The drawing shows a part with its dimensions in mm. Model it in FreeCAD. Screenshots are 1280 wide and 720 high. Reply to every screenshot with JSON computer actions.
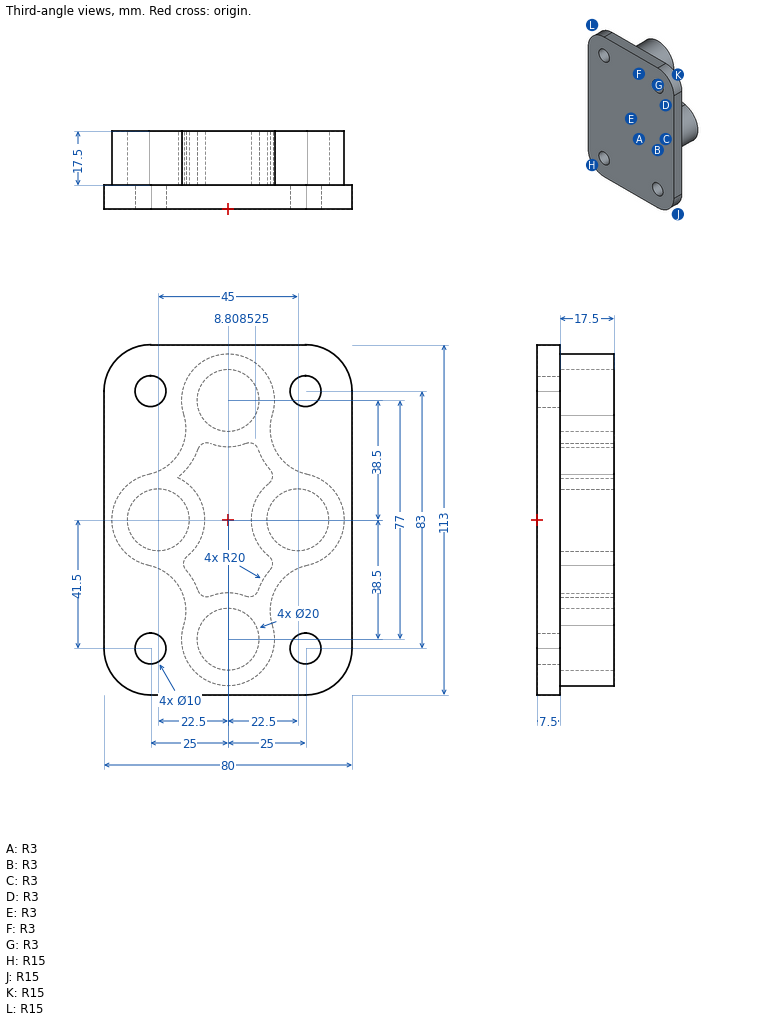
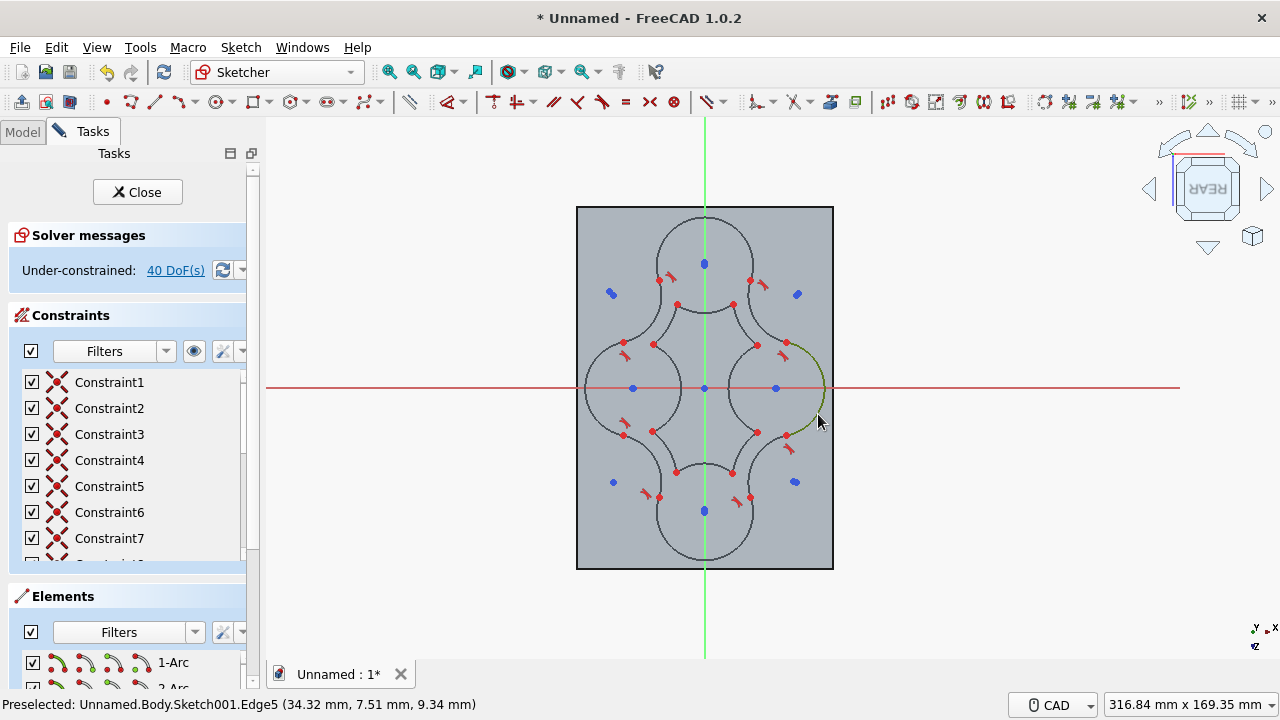
{"action": "left_click", "coordinate": [734, 368]}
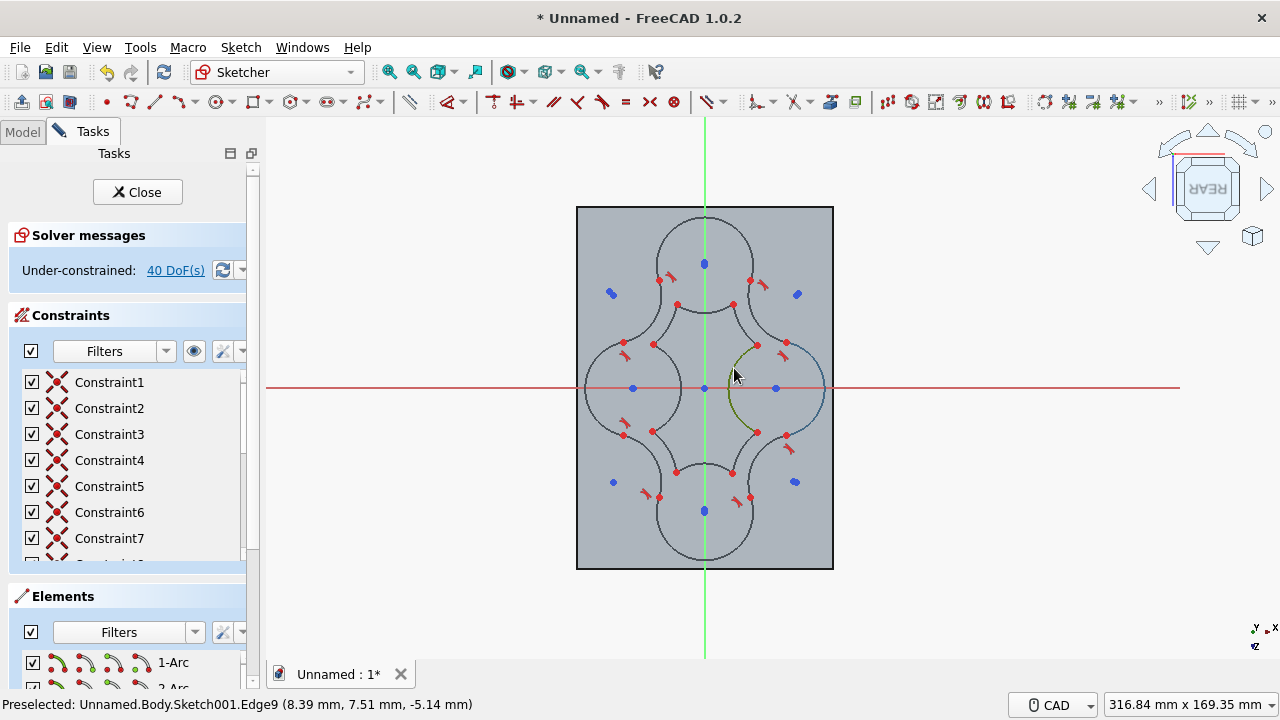
{"action": "key", "text": "c"}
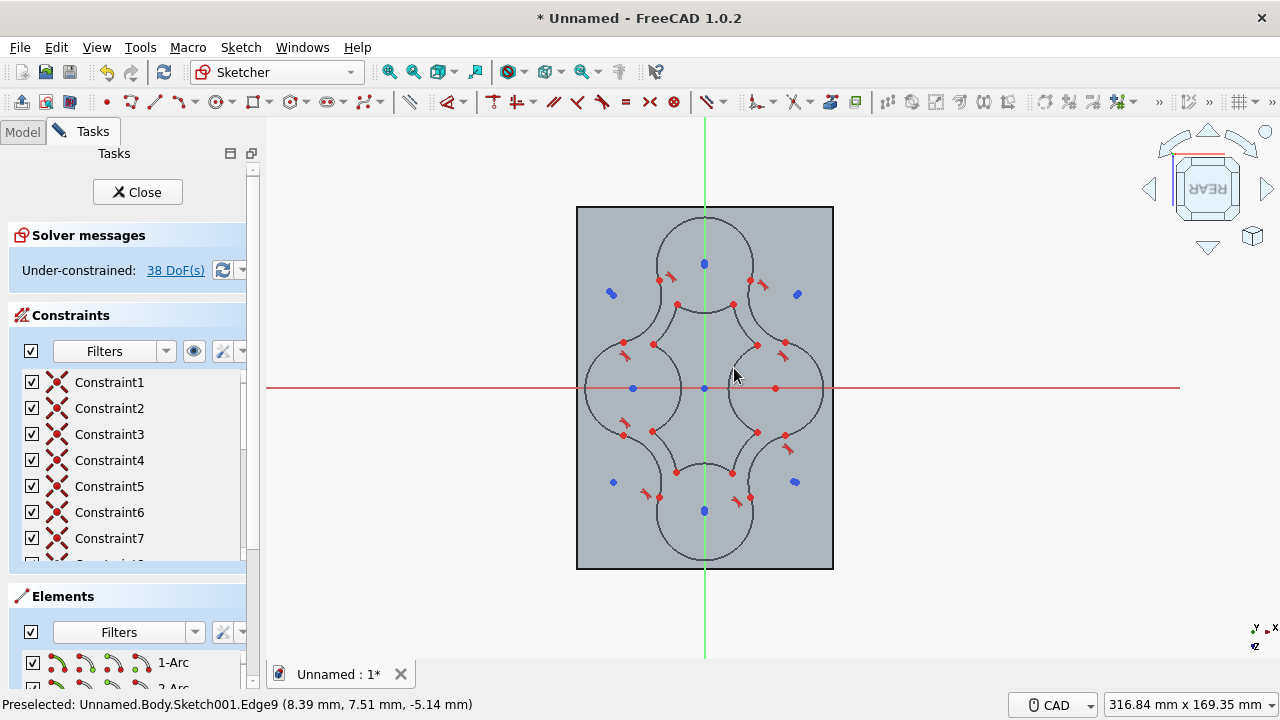
{"action": "left_click", "coordinate": [765, 446]}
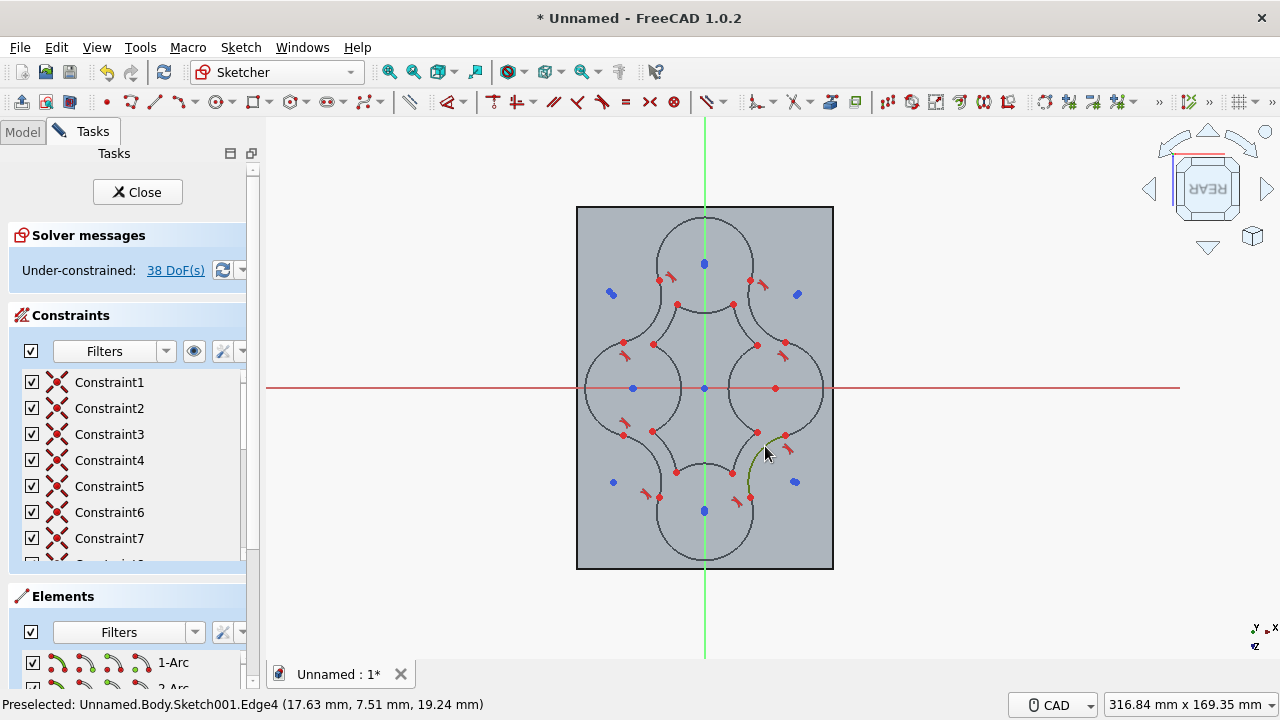
{"action": "left_click", "coordinate": [747, 442]}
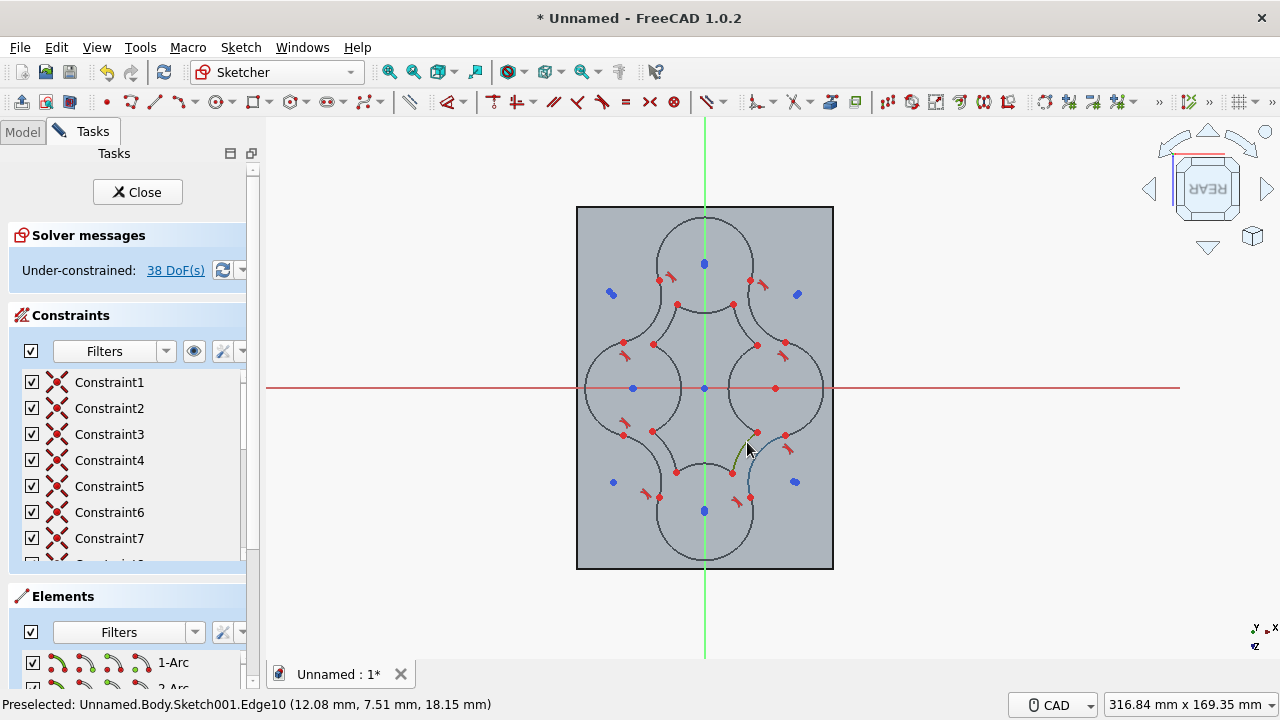
{"action": "key", "text": "c"}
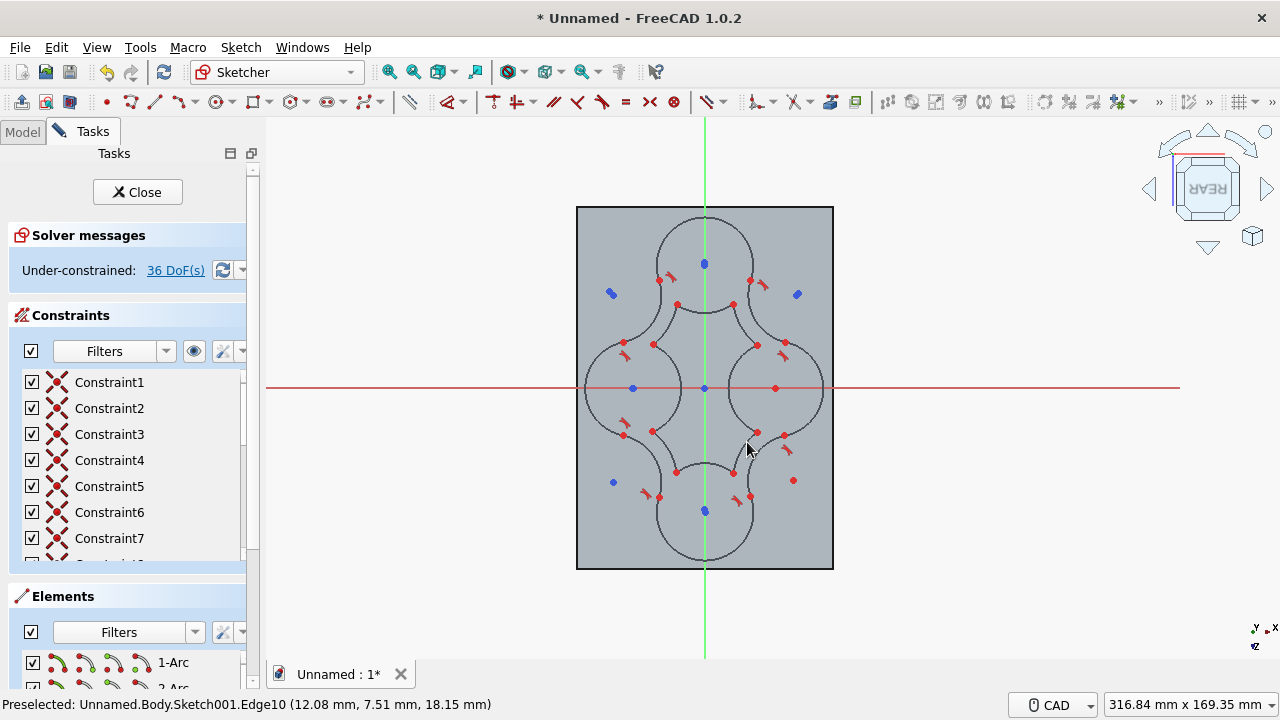
{"action": "left_click", "coordinate": [672, 548]}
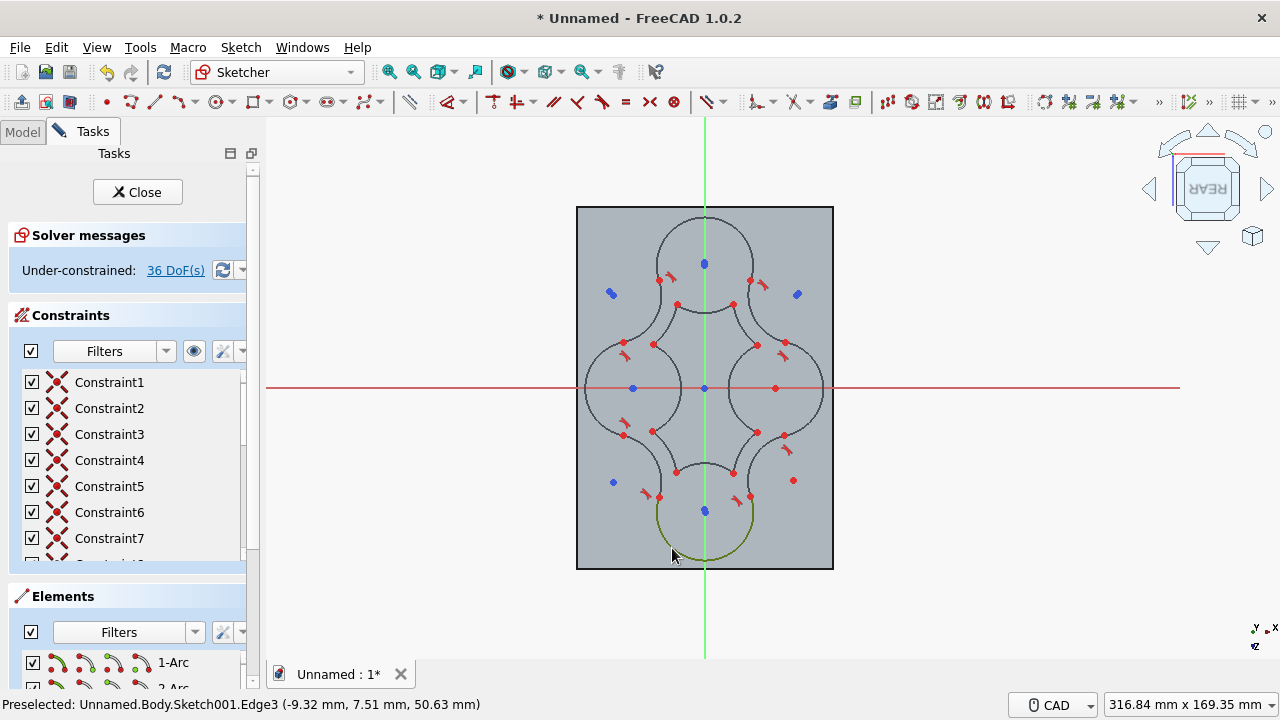
{"action": "left_click", "coordinate": [717, 465]}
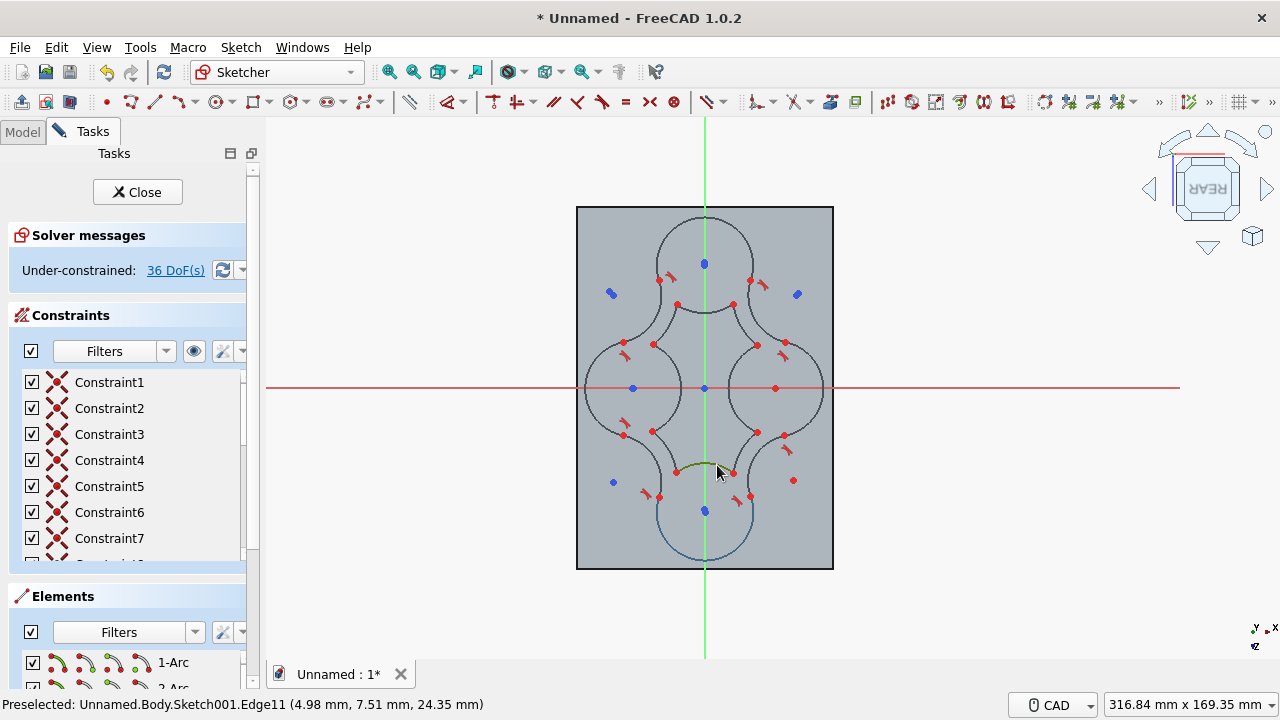
{"action": "key", "text": "c"}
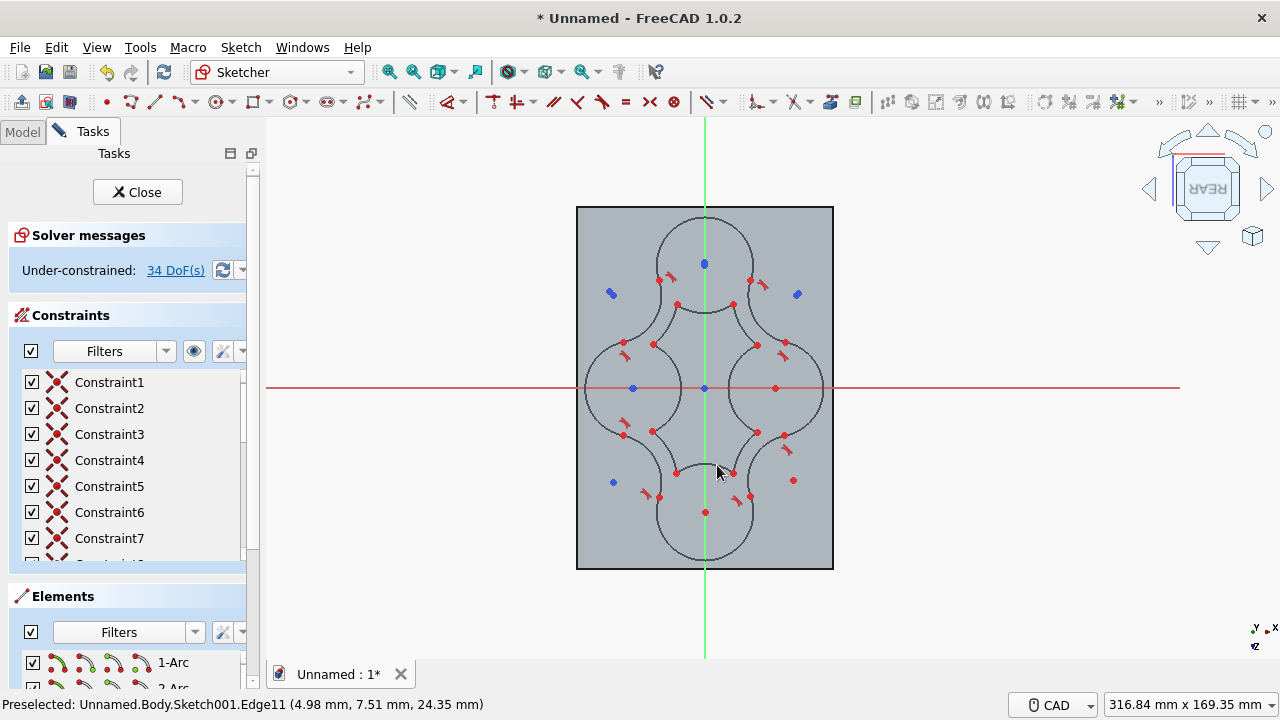
{"action": "left_click", "coordinate": [661, 473]}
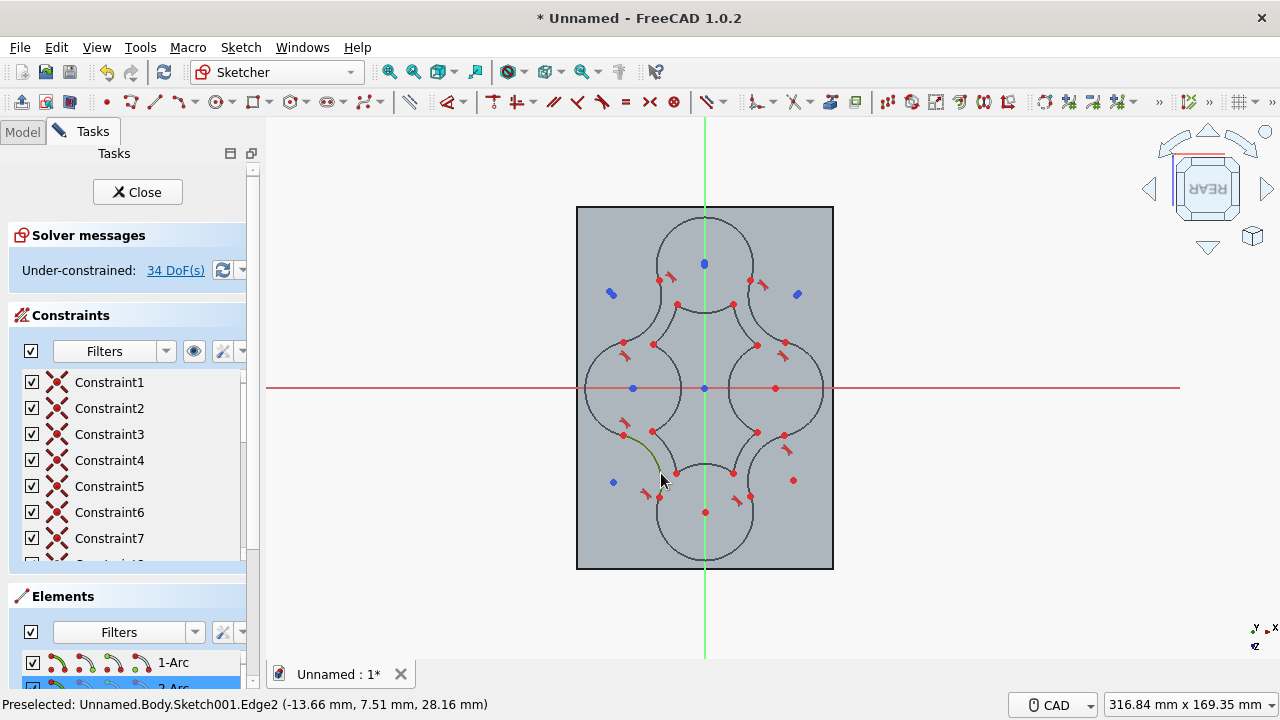
{"action": "left_click", "coordinate": [673, 459]}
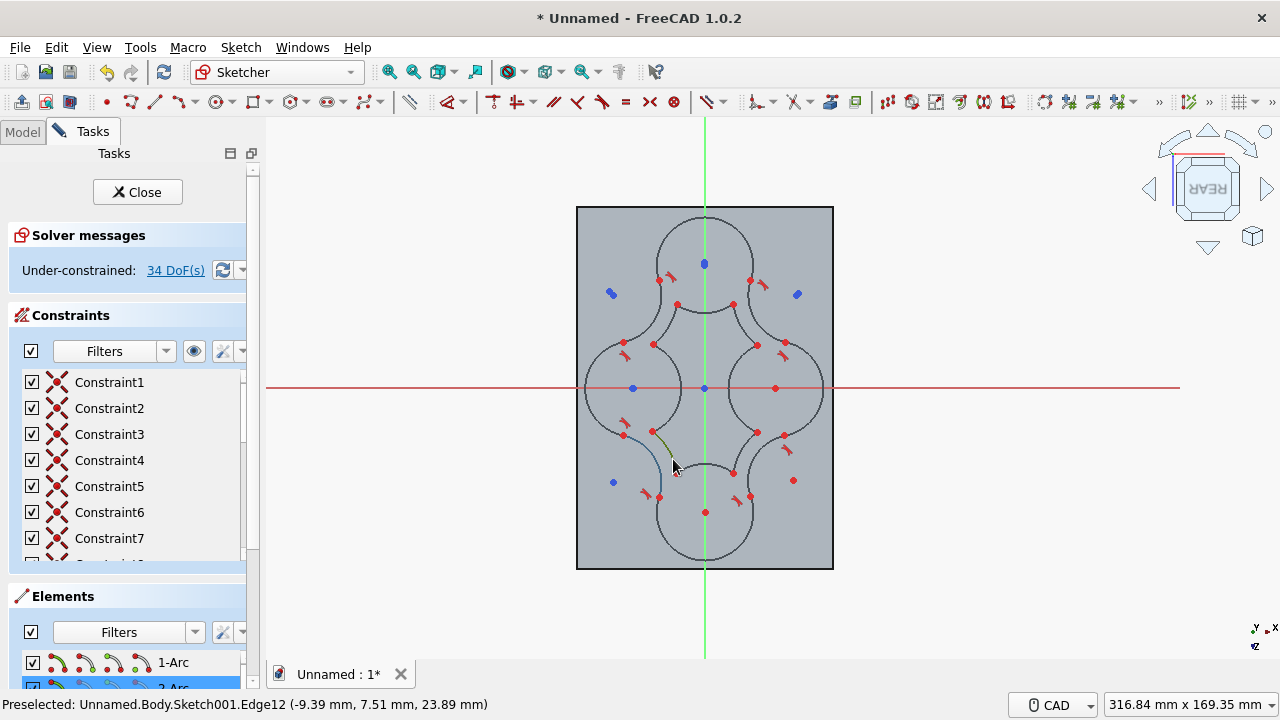
{"action": "left_click", "coordinate": [494, 102]}